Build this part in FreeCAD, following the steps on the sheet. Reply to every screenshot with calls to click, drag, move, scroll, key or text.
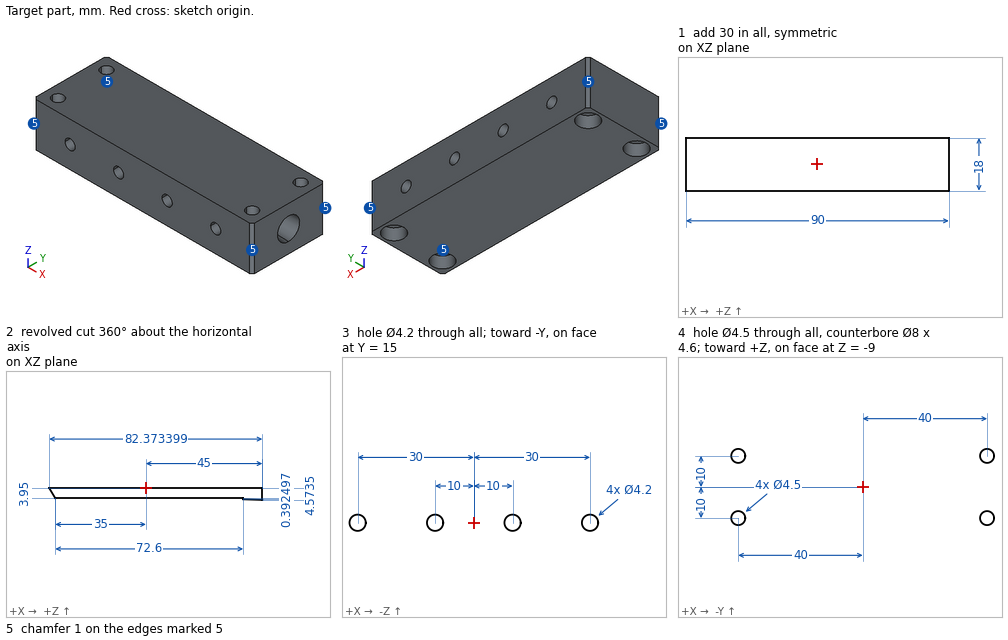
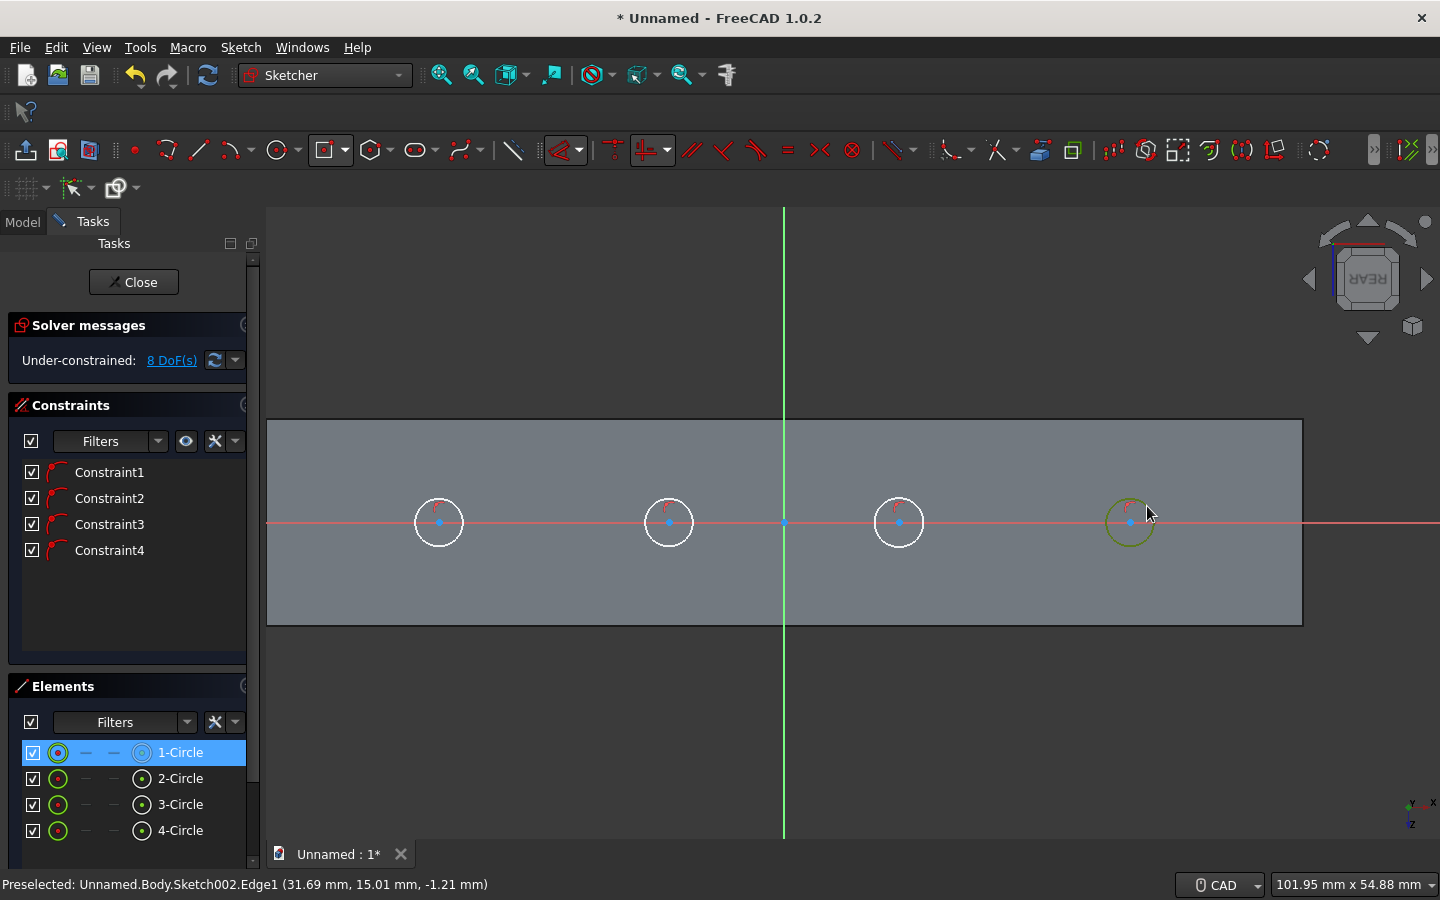
click(916, 505)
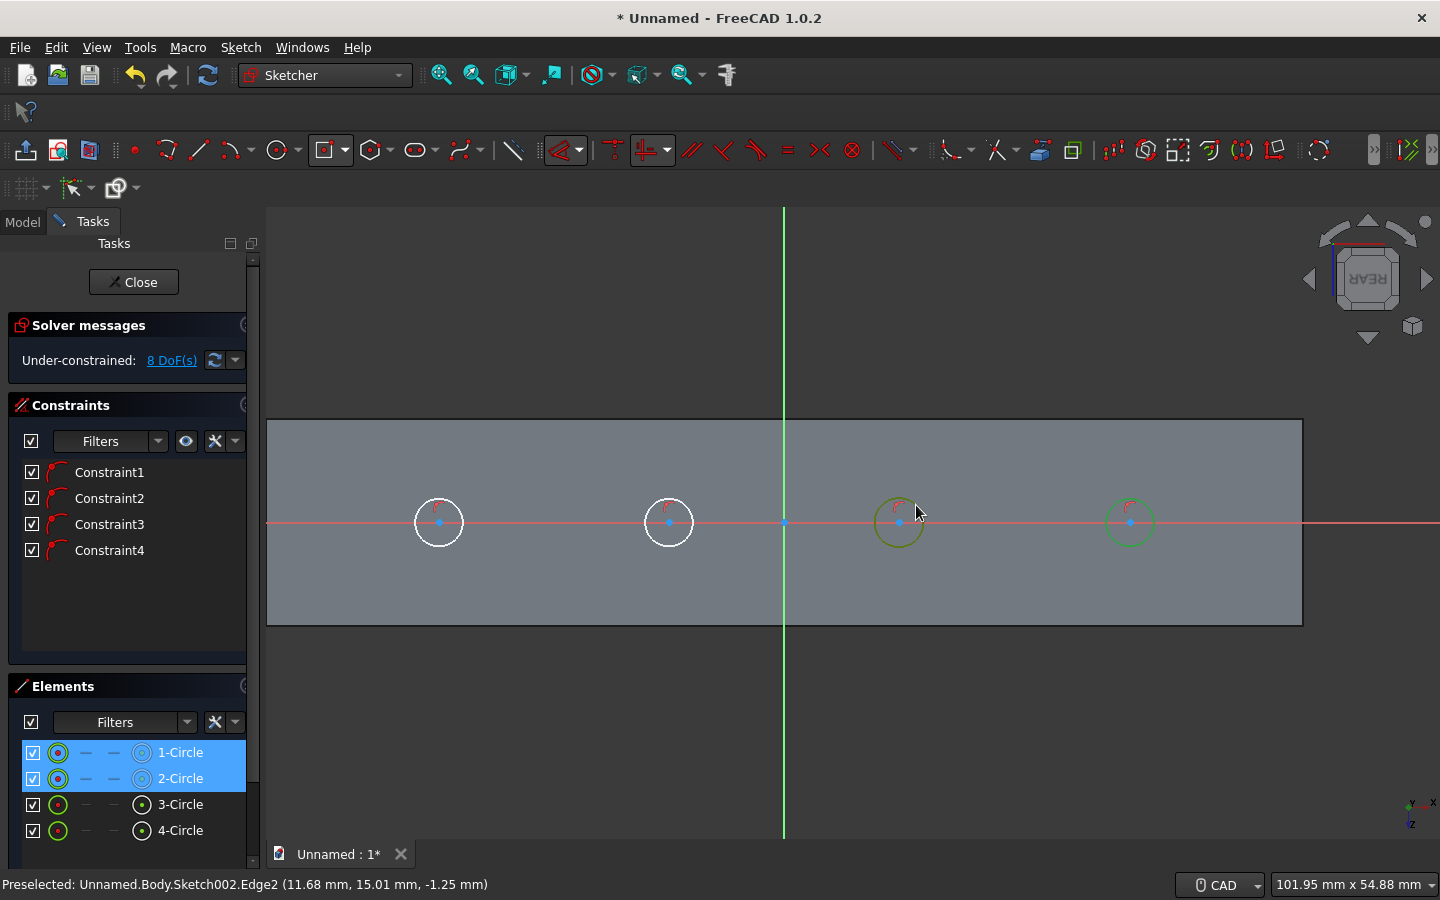
click(686, 506)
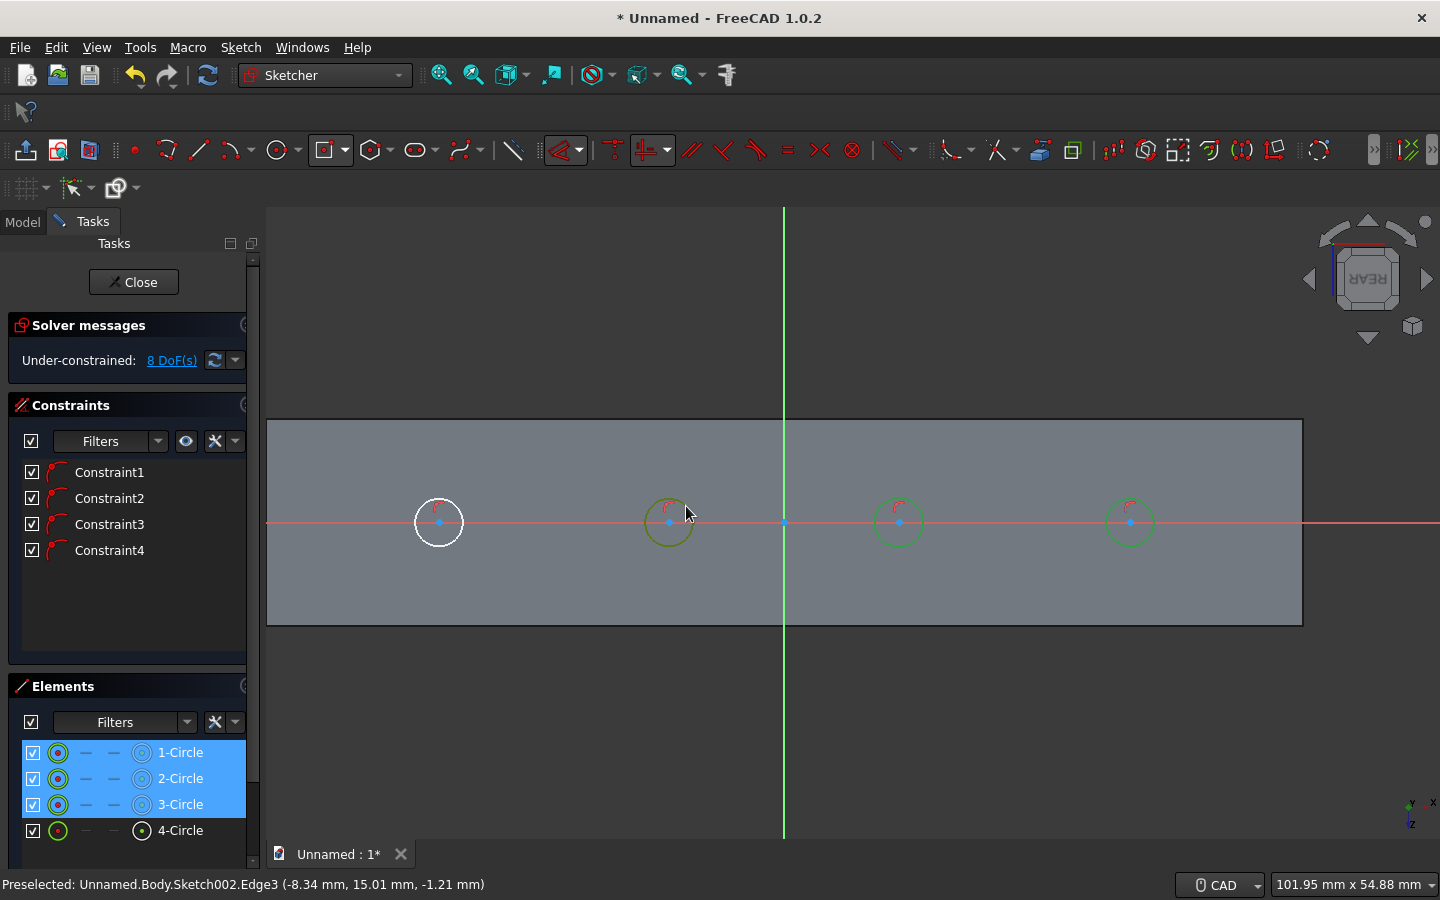
click(456, 506)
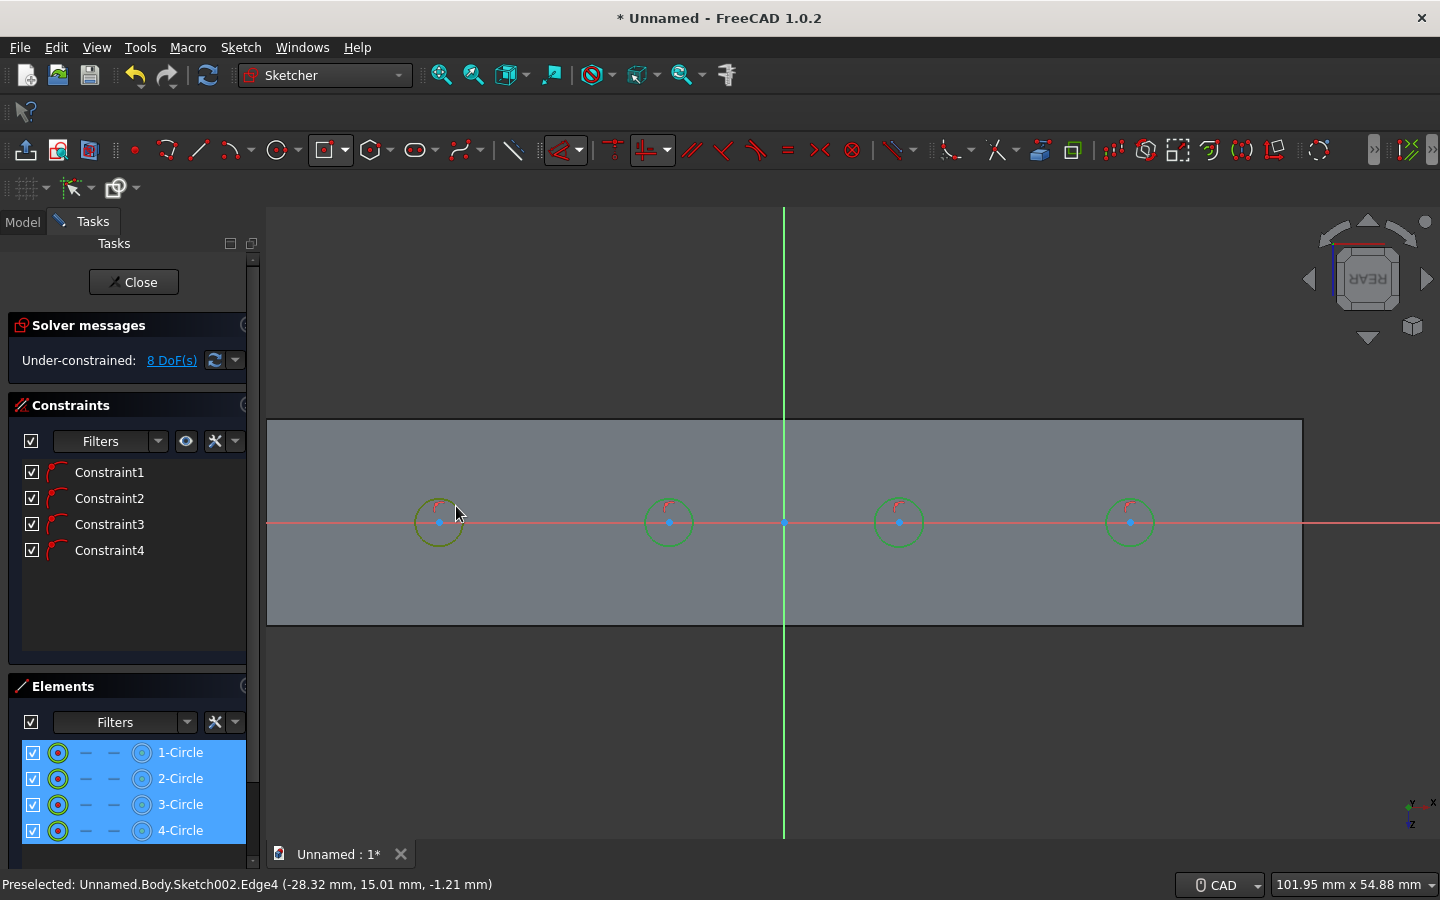
click(788, 150)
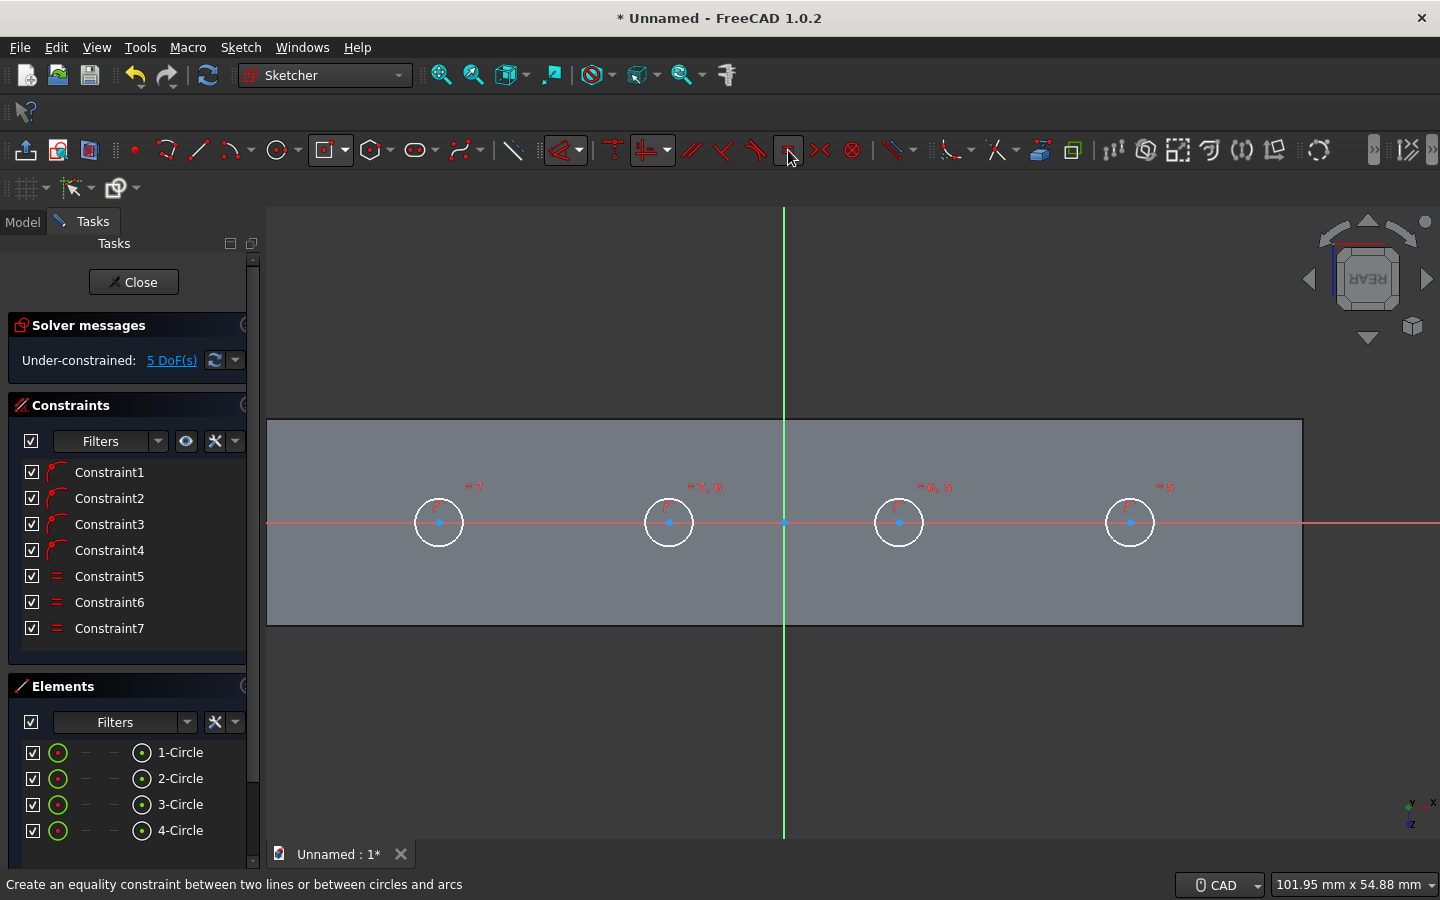
click(1147, 506)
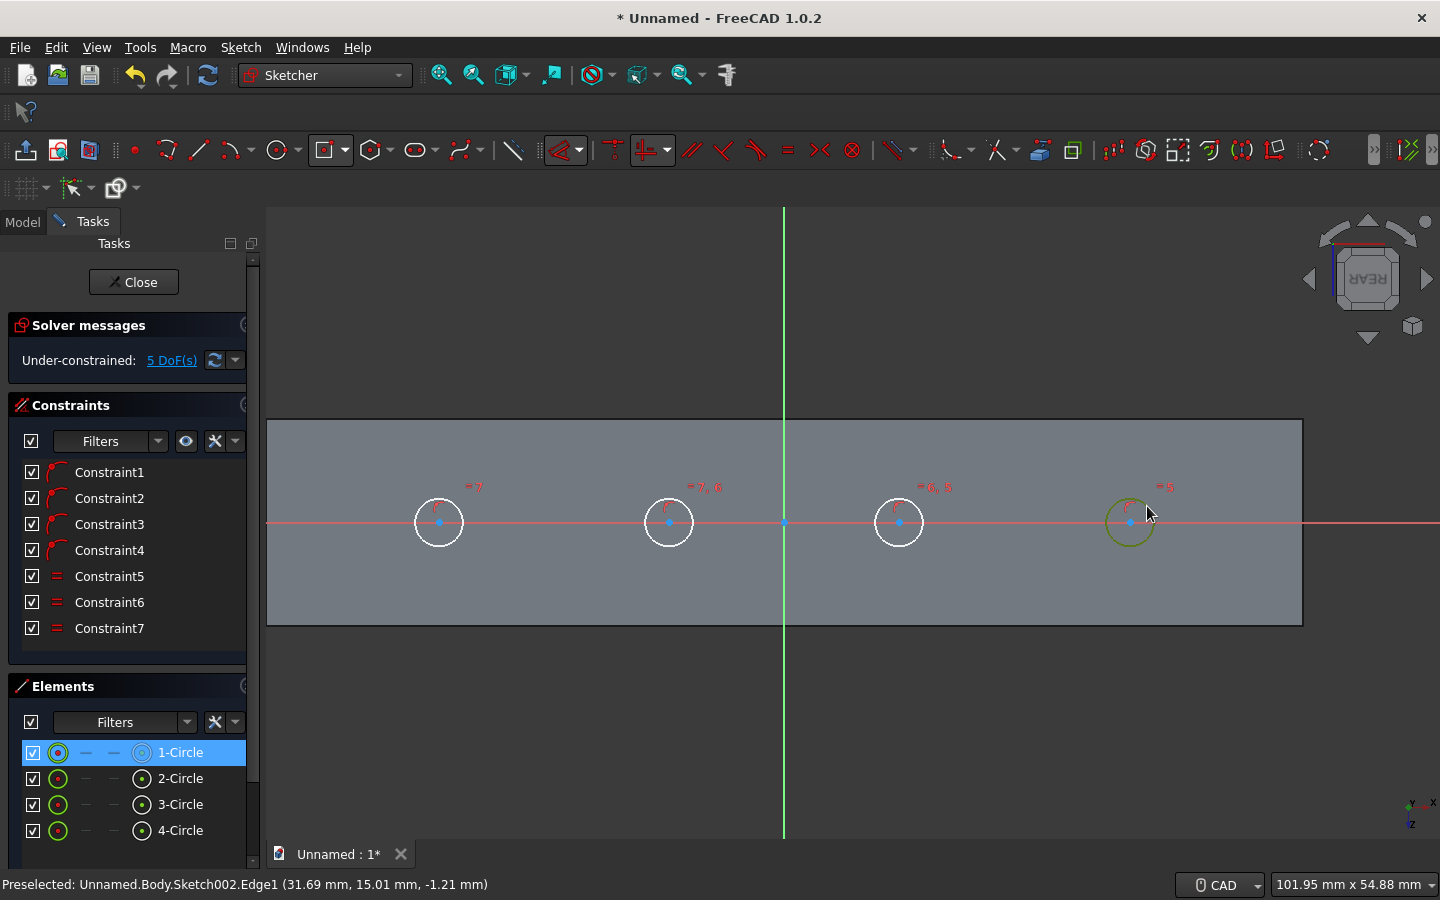
click(582, 150)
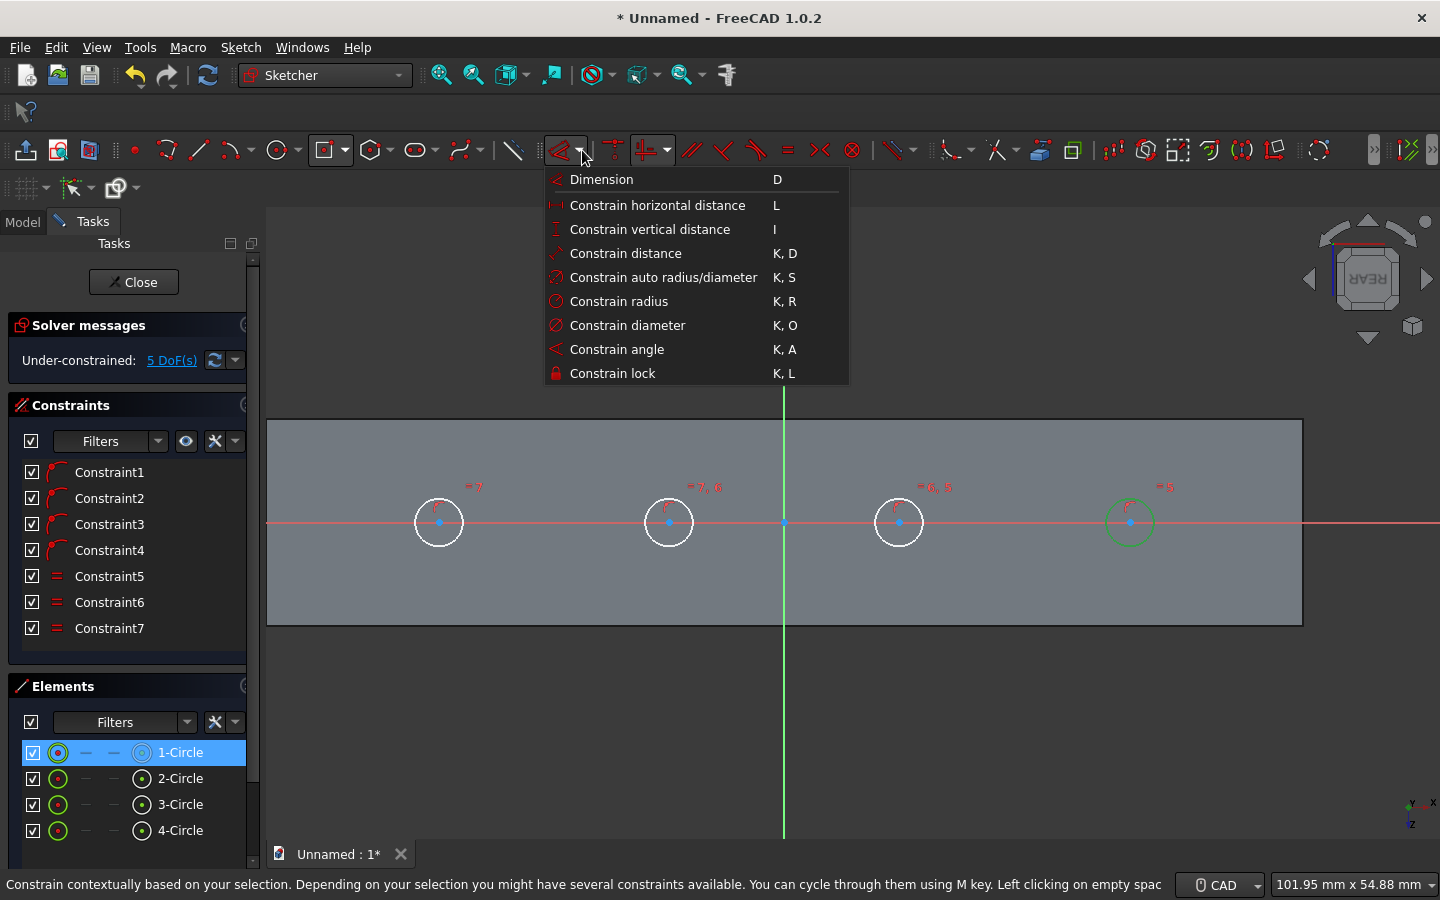
click(697, 325)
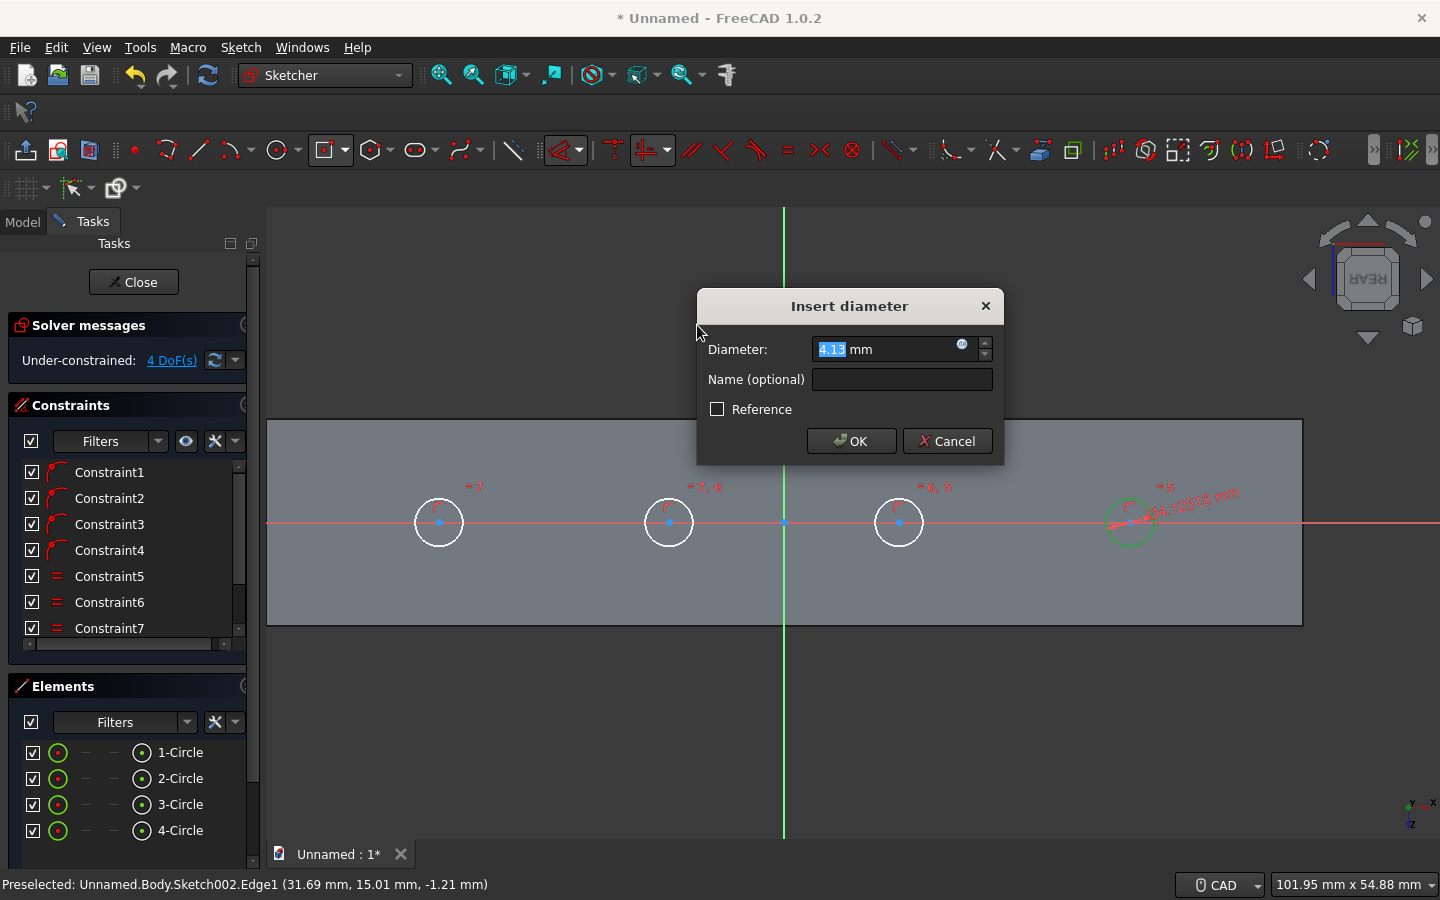
text(4.2)
key(Return)